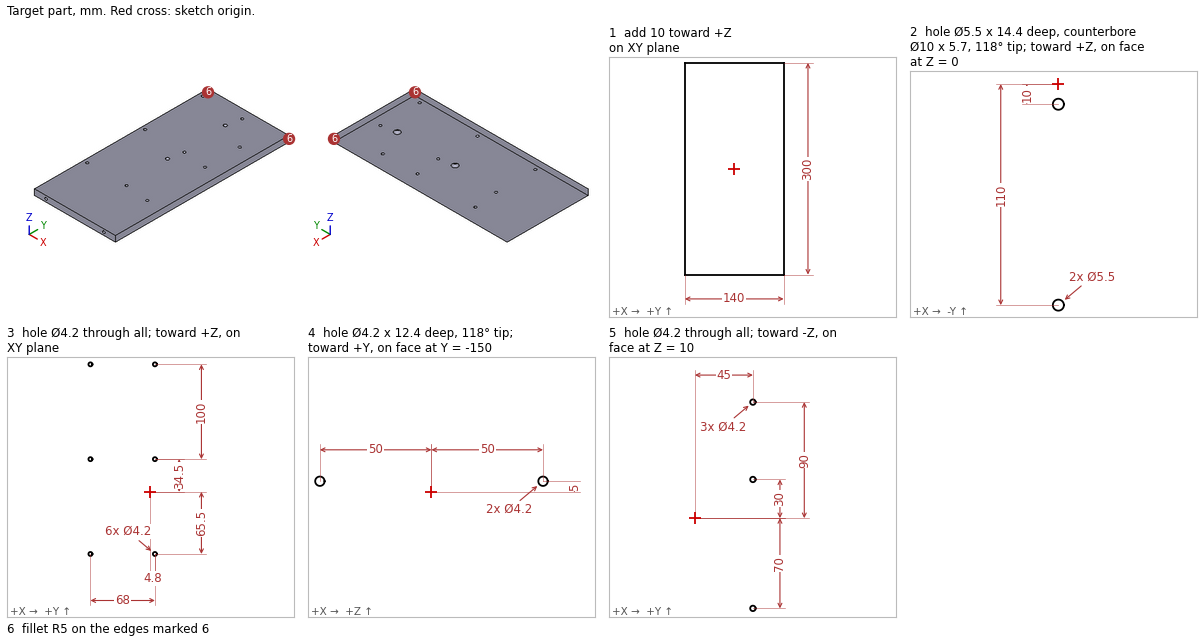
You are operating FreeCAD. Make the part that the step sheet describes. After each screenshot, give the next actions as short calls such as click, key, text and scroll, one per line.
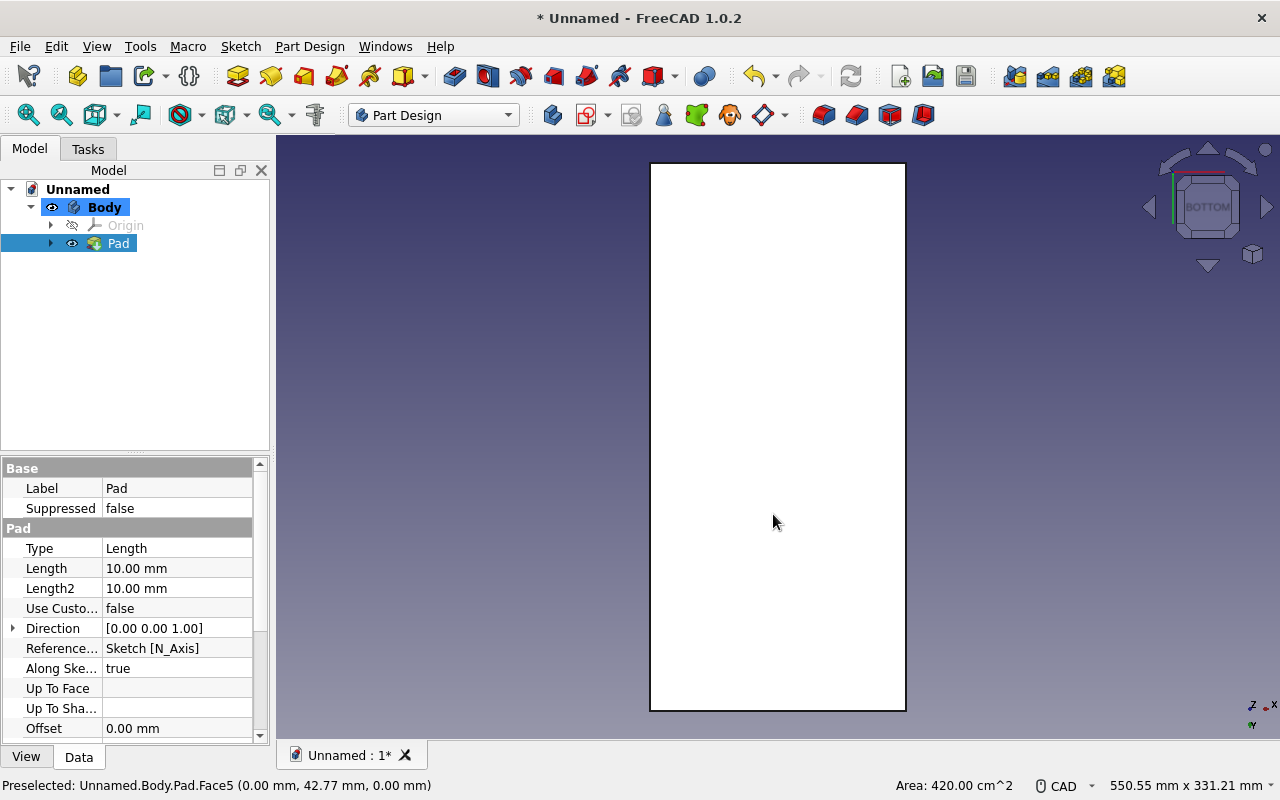
click(586, 116)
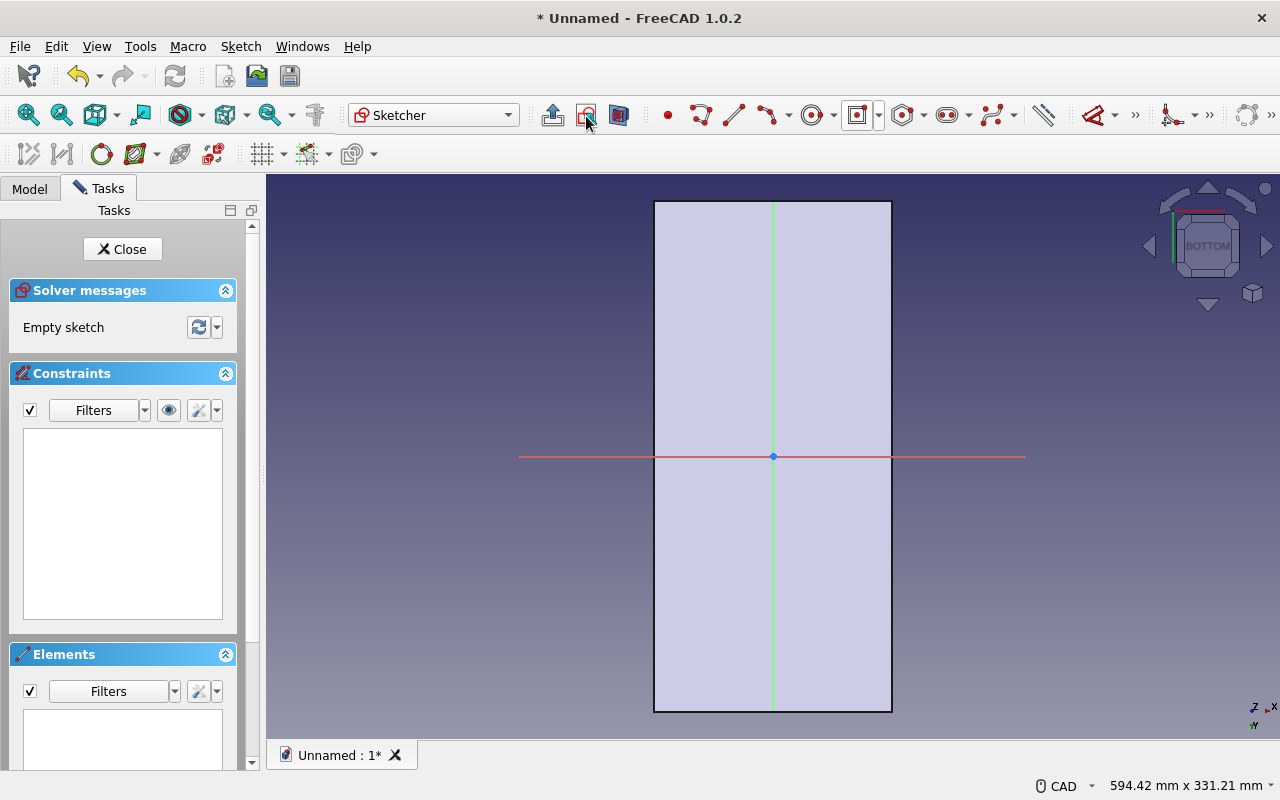
scroll(856, 670, up, 3)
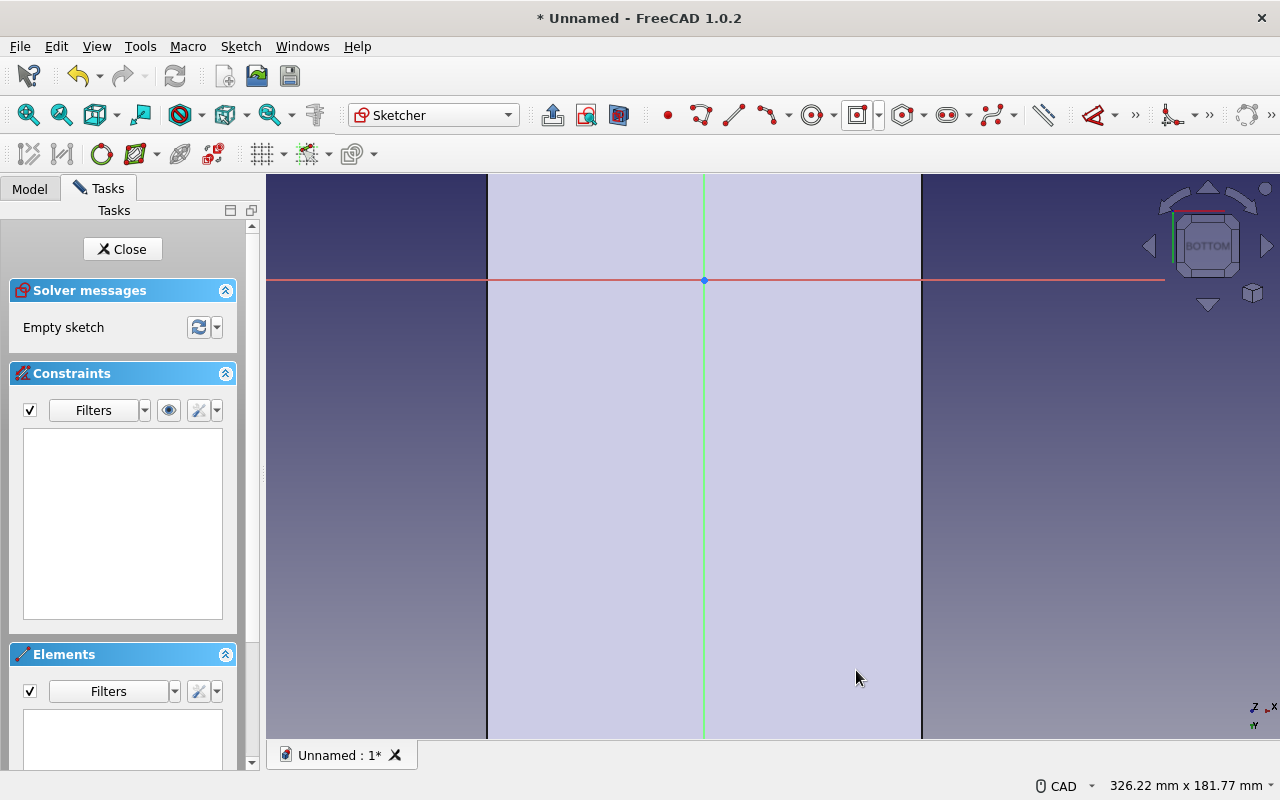
click(812, 116)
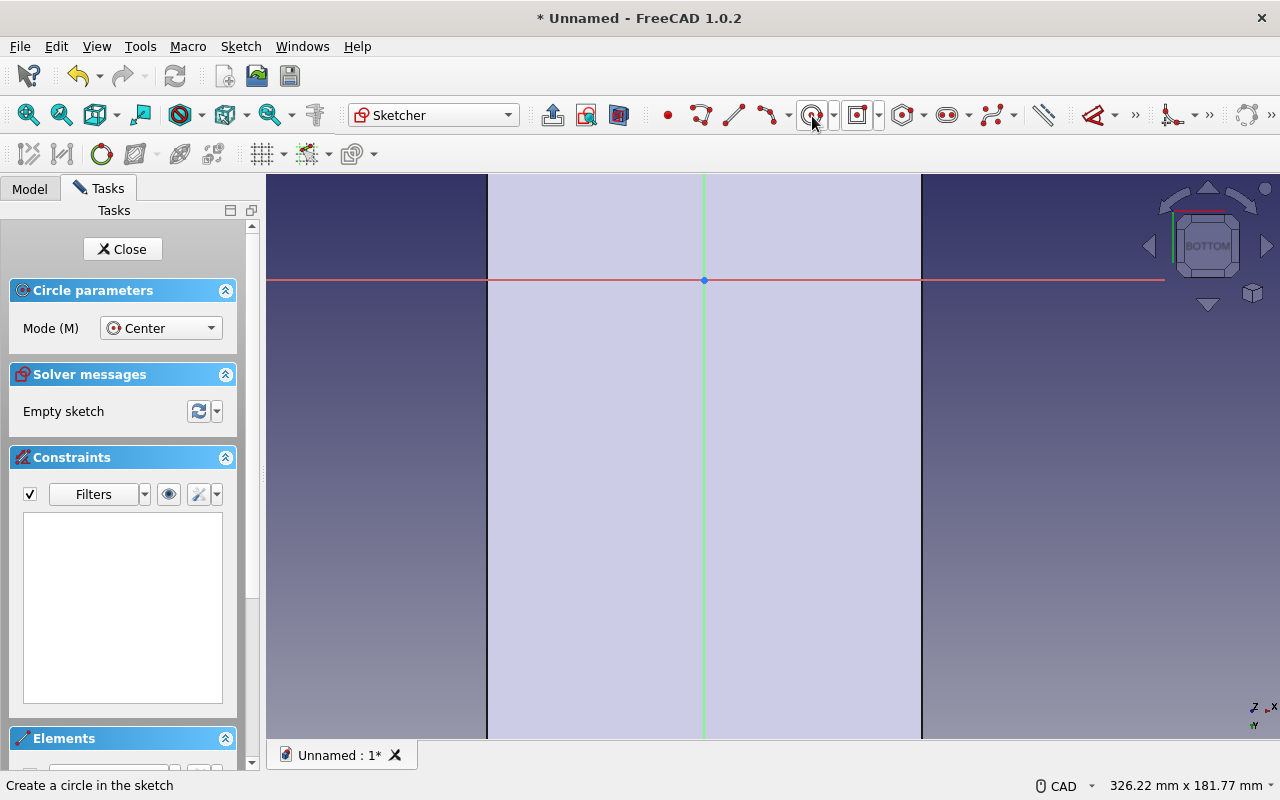
scroll(704, 622, up, 5)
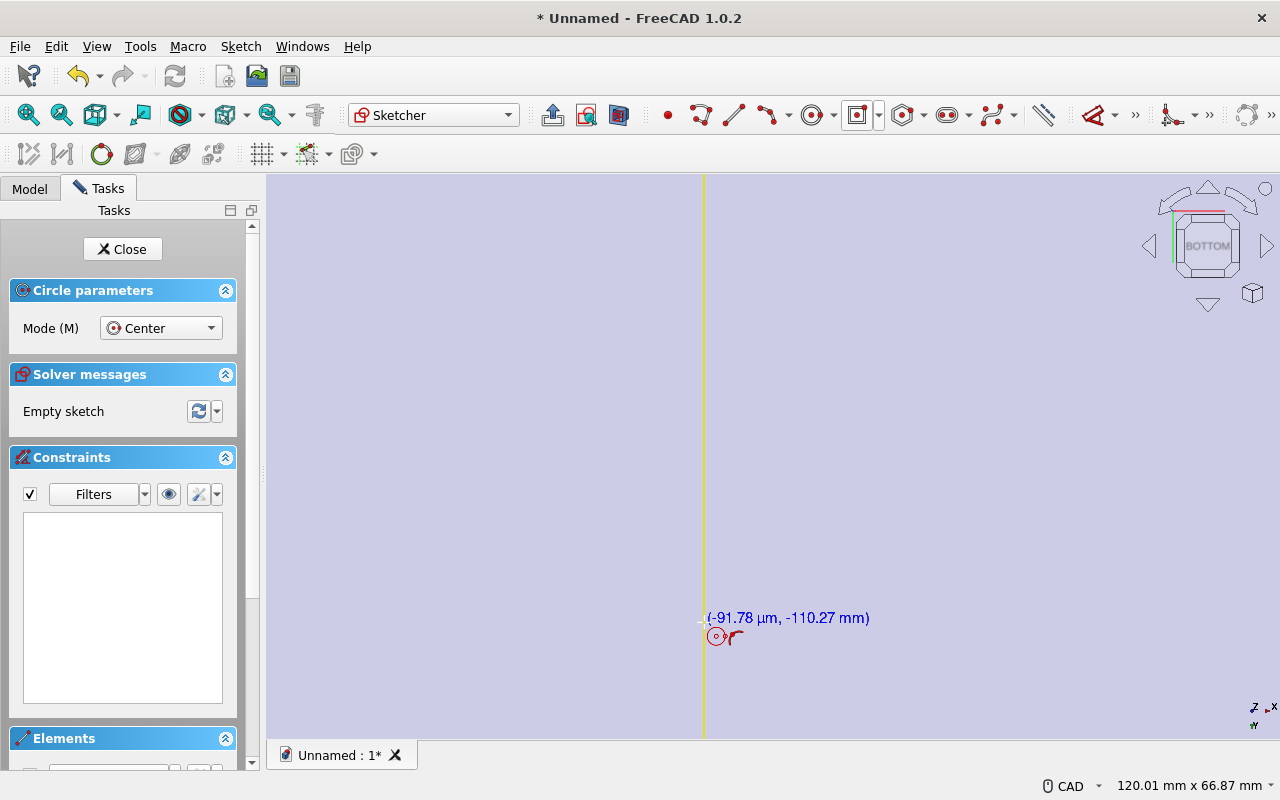
click(704, 621)
click(720, 605)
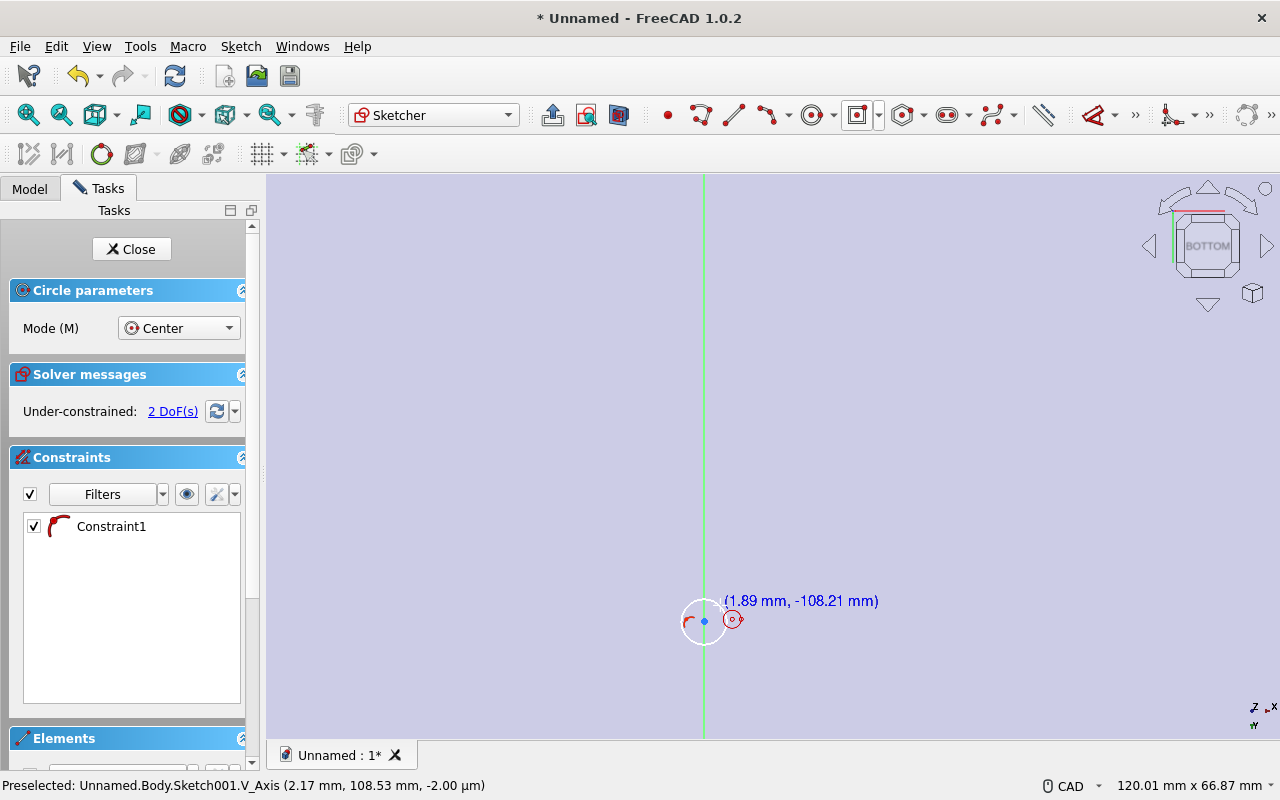
scroll(705, 624, down, 5)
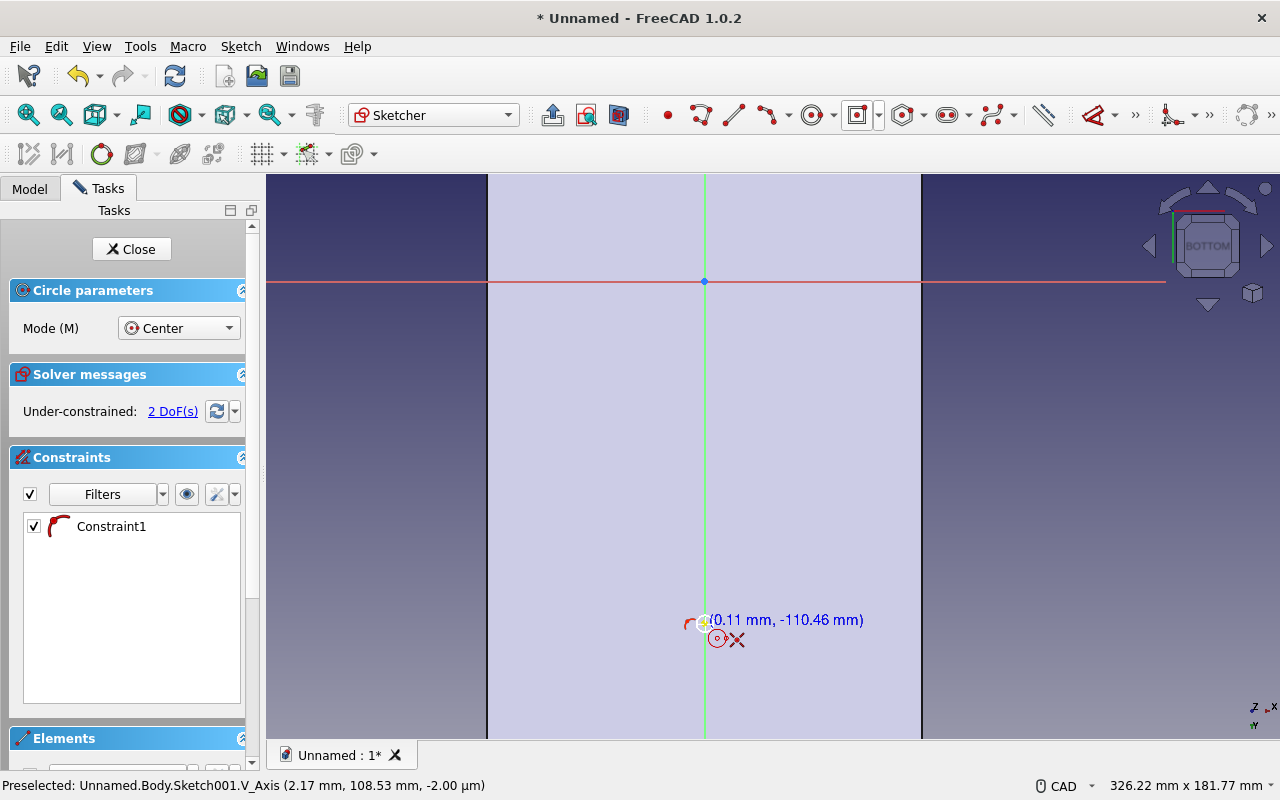
scroll(705, 313, up, 5)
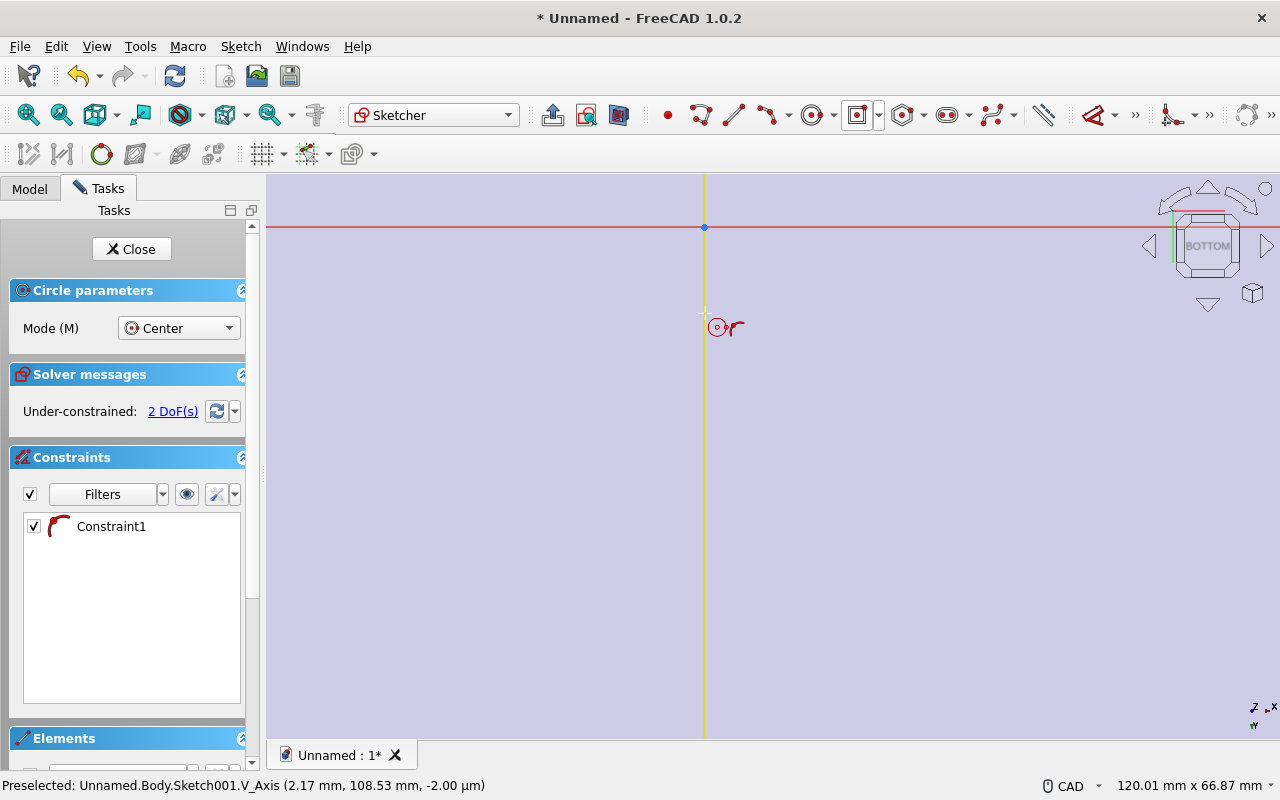
click(704, 312)
click(720, 295)
key(Escape)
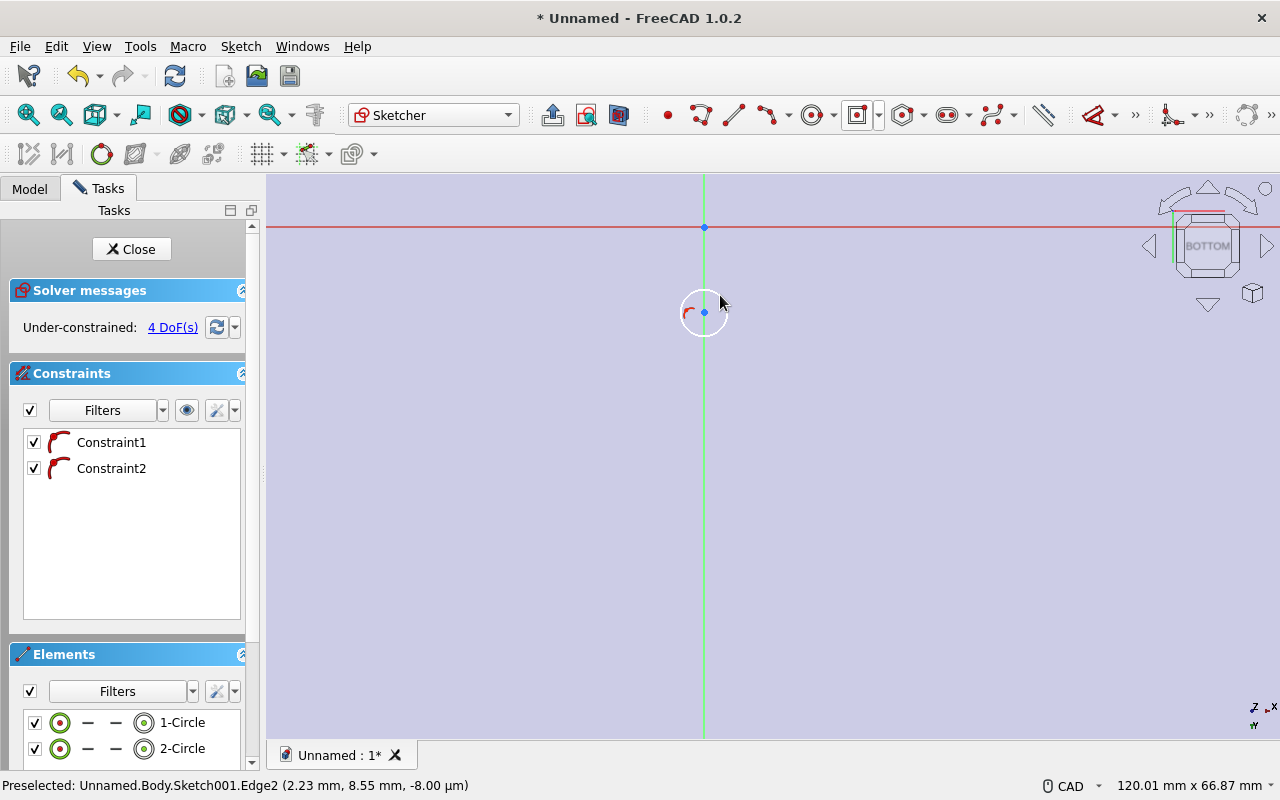
scroll(705, 313, down, 5)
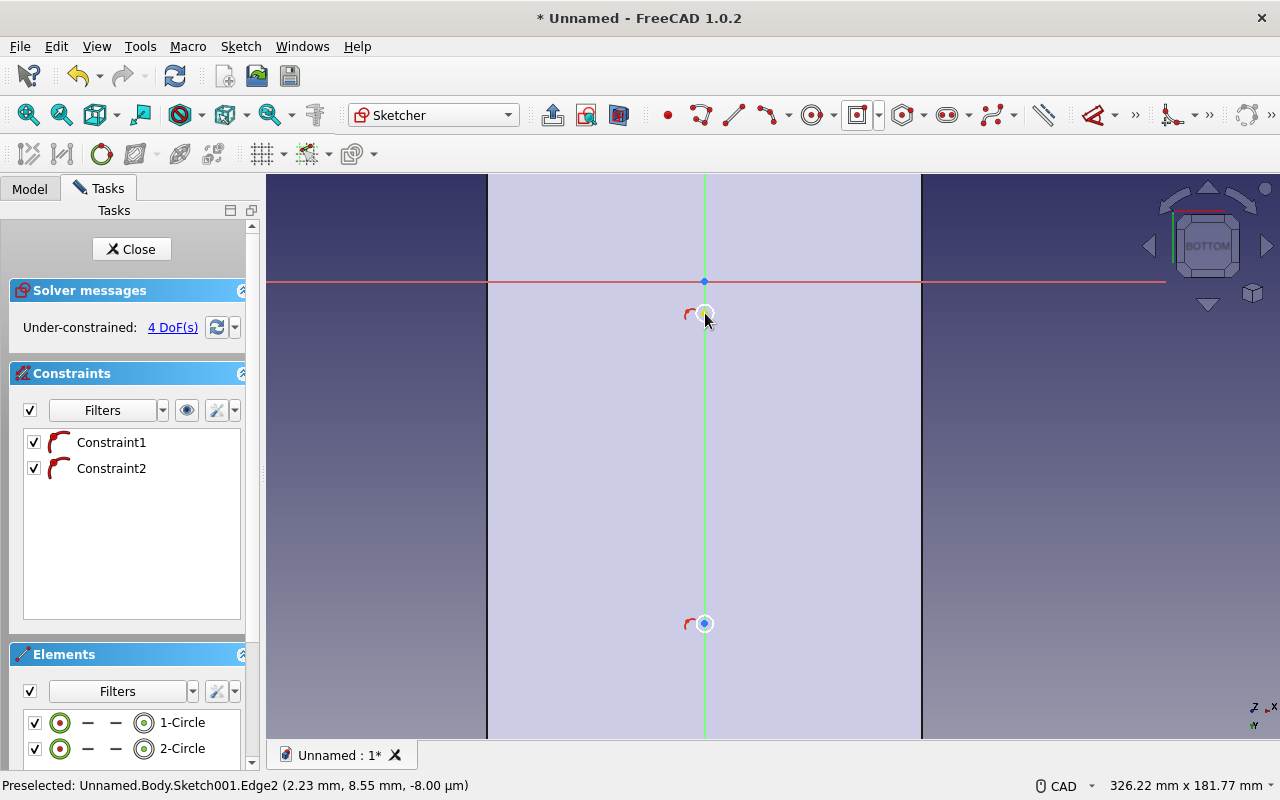
scroll(711, 618, up, 5)